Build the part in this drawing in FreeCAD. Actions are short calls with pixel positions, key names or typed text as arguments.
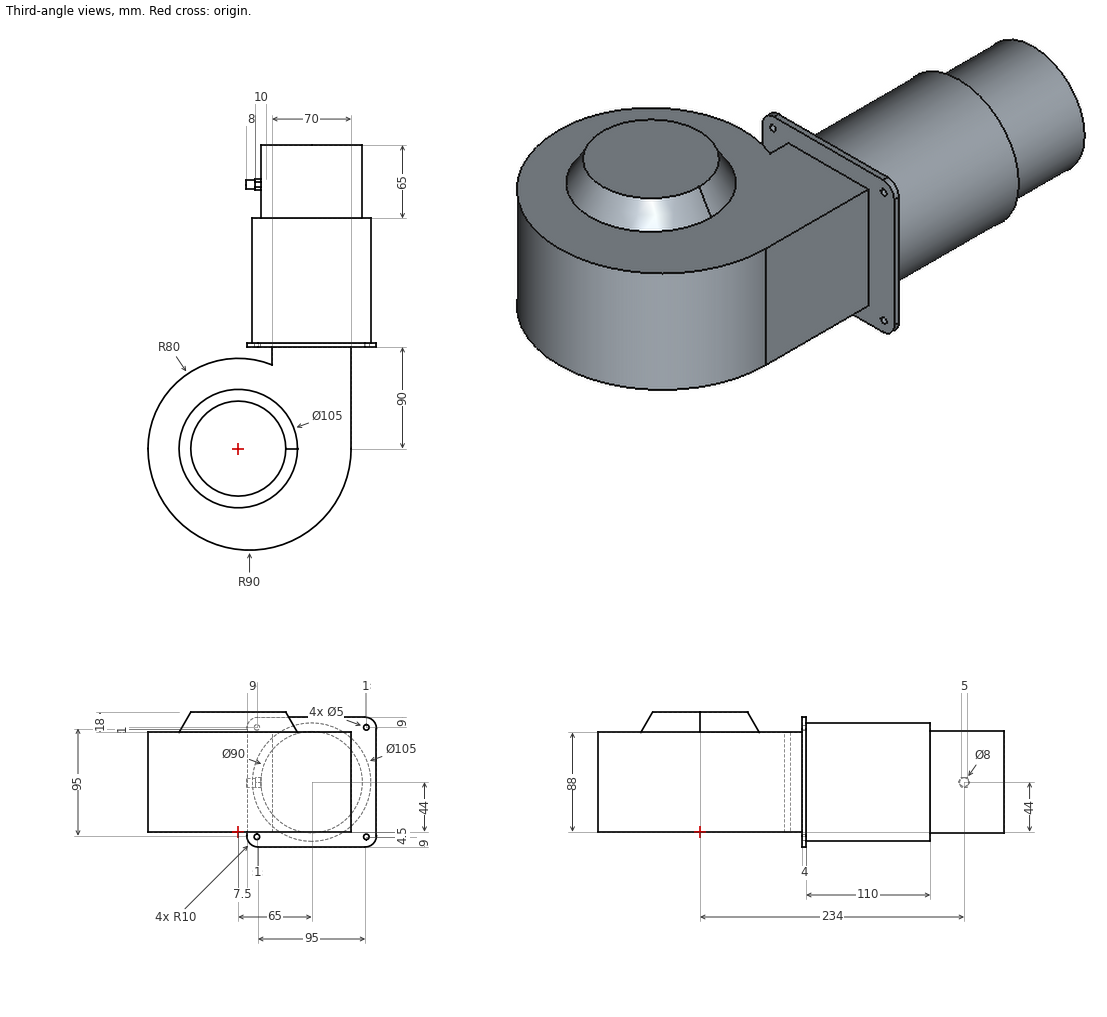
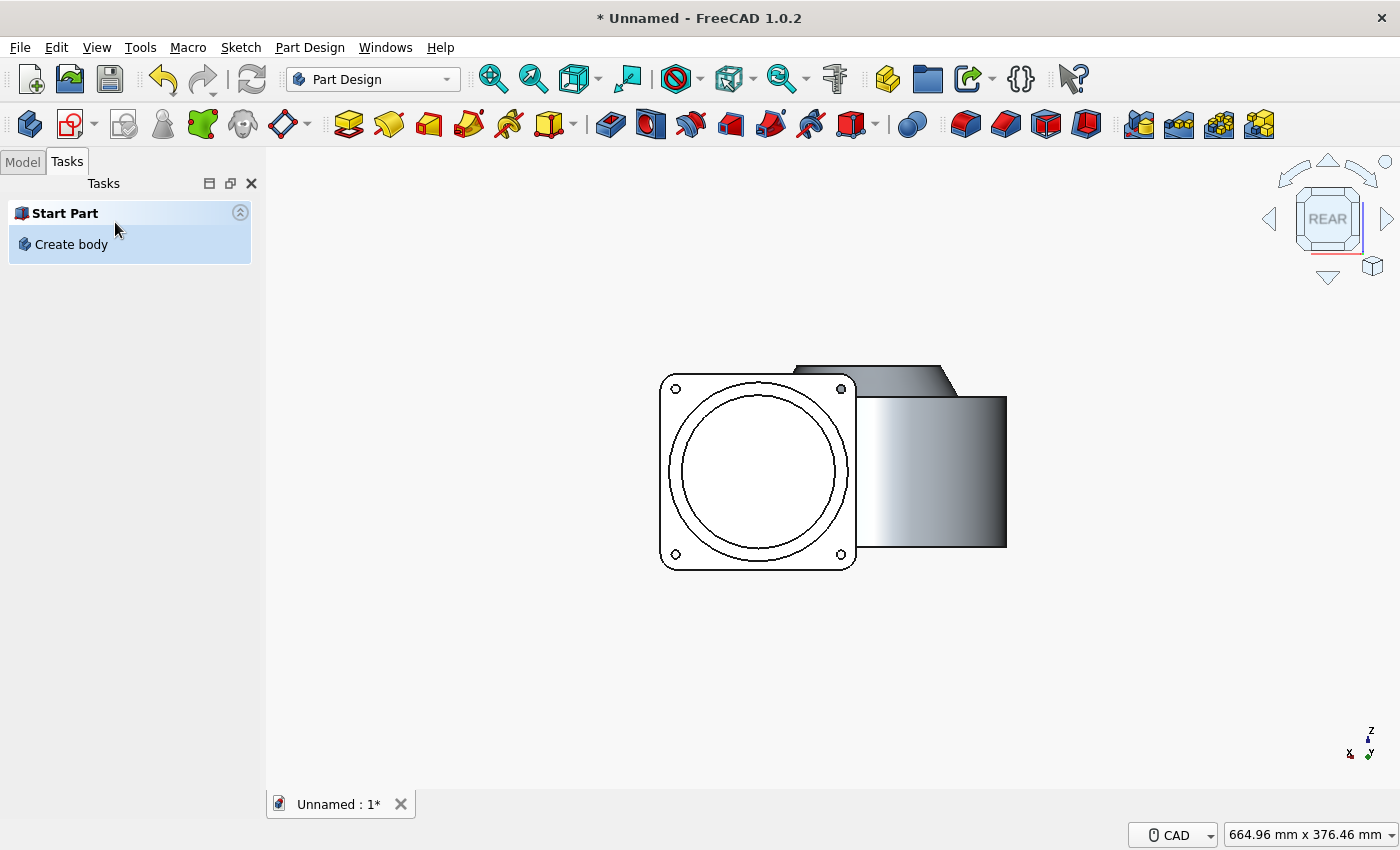
key(v)
key(f)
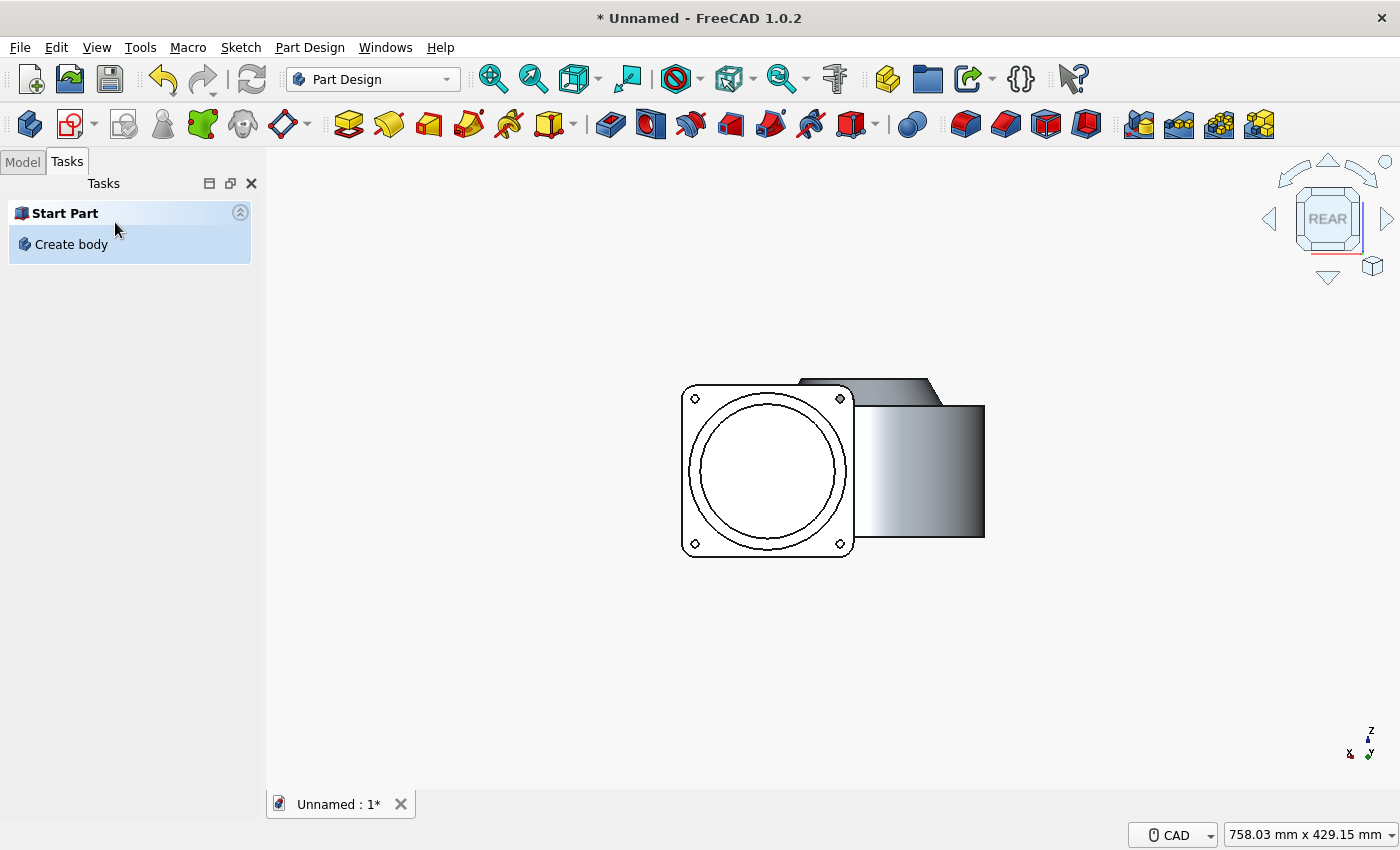
click(30, 124)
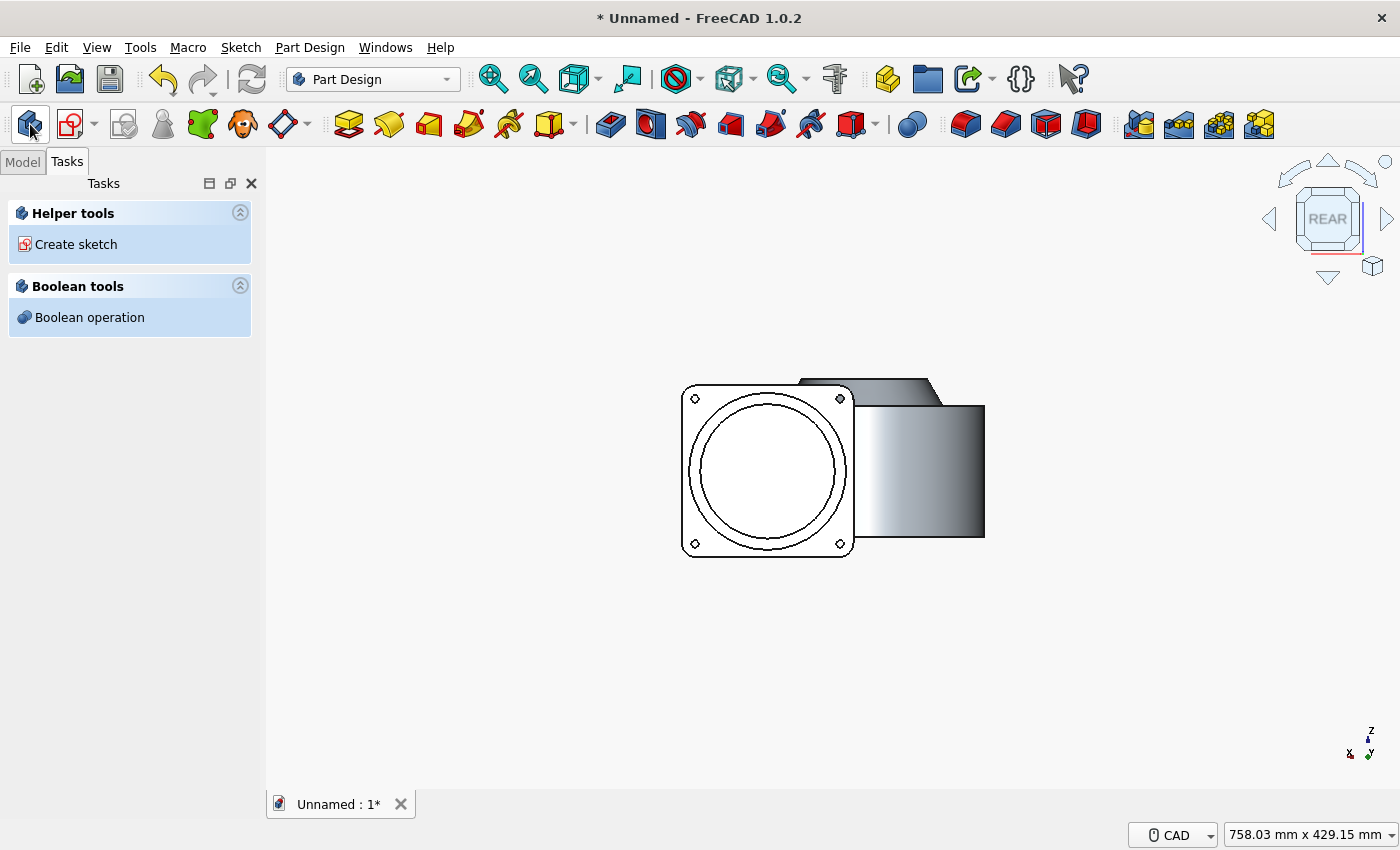
click(23, 161)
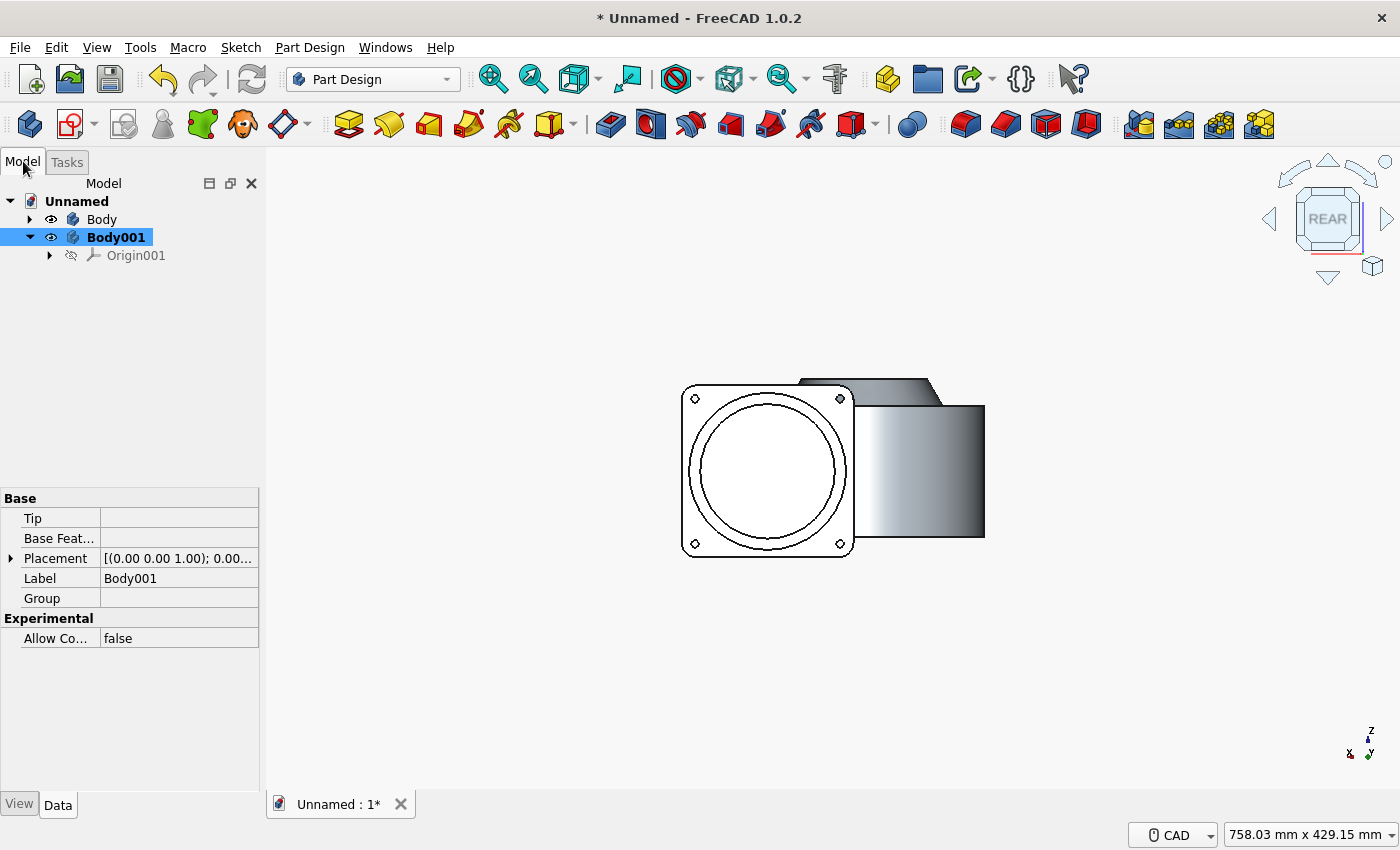
click(50, 255)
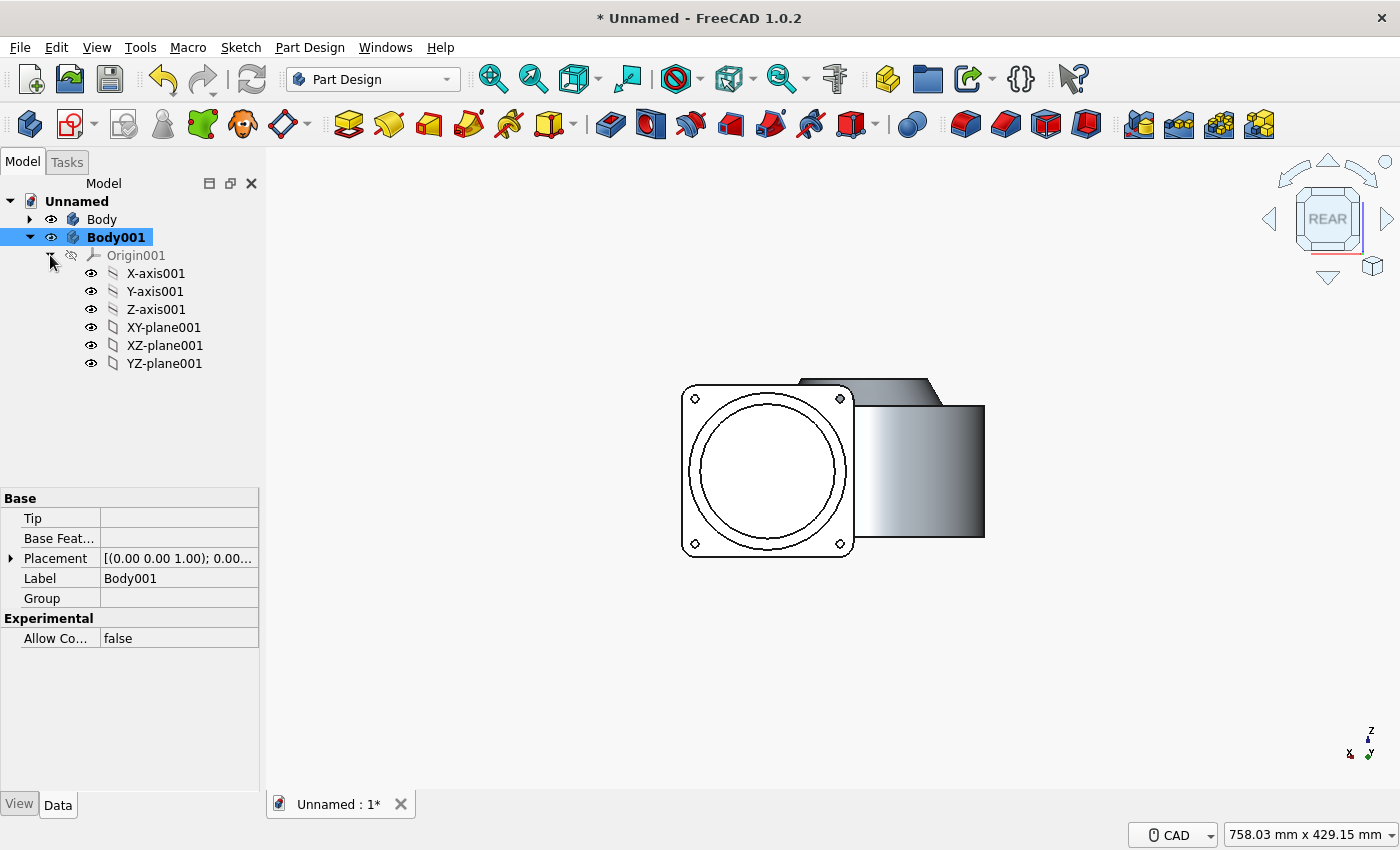
click(136, 363)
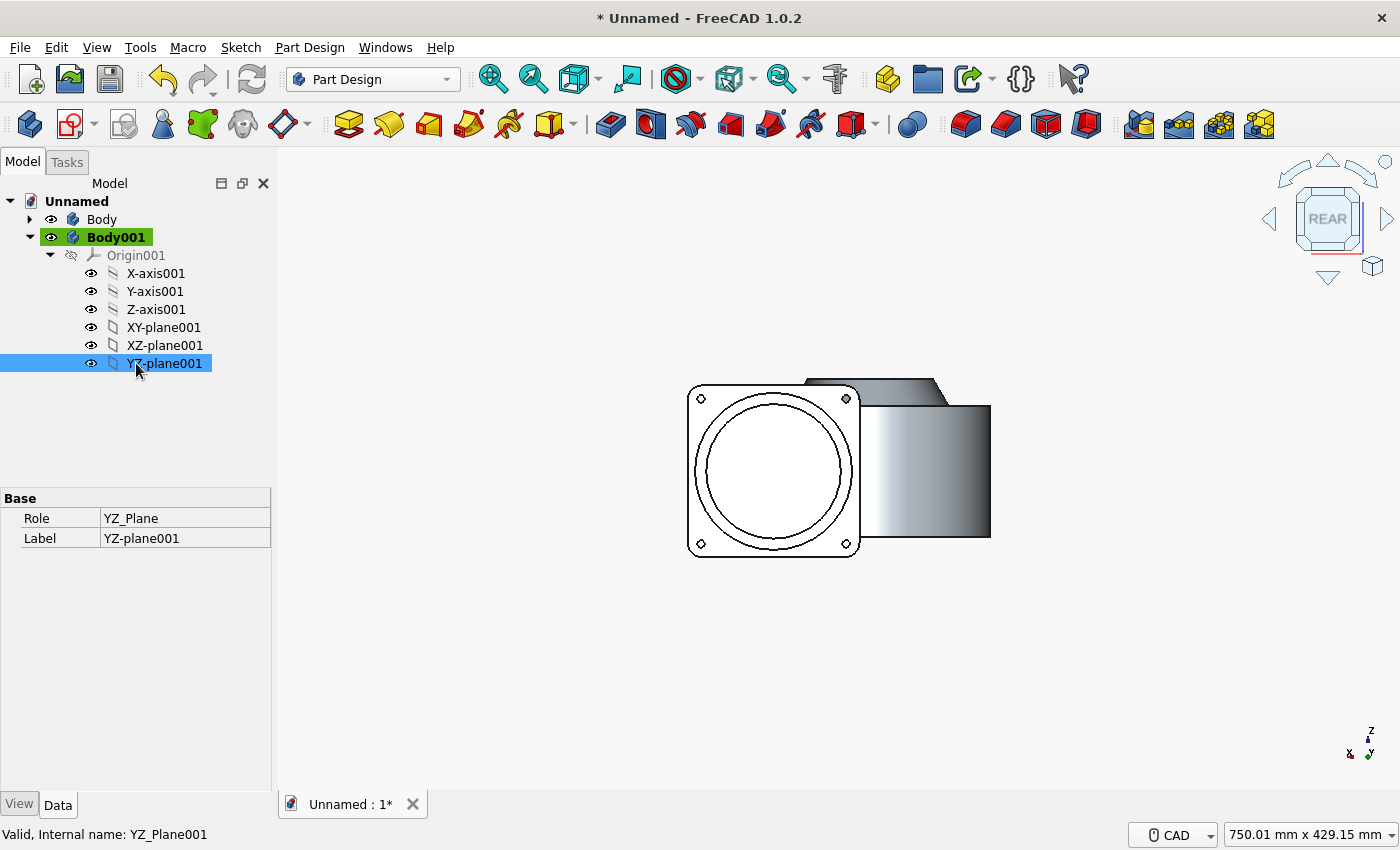
click(284, 124)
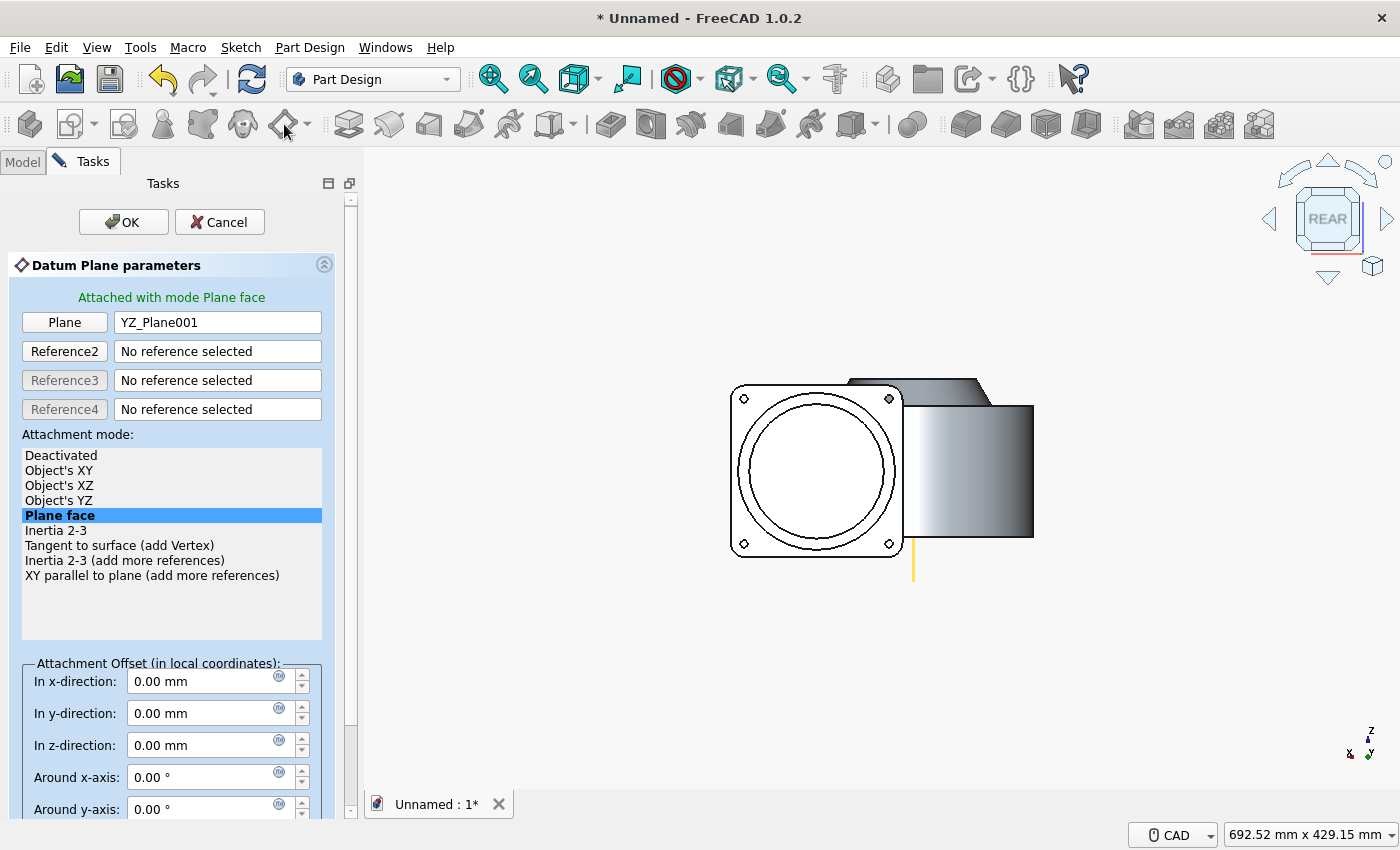
triple_click(210, 745)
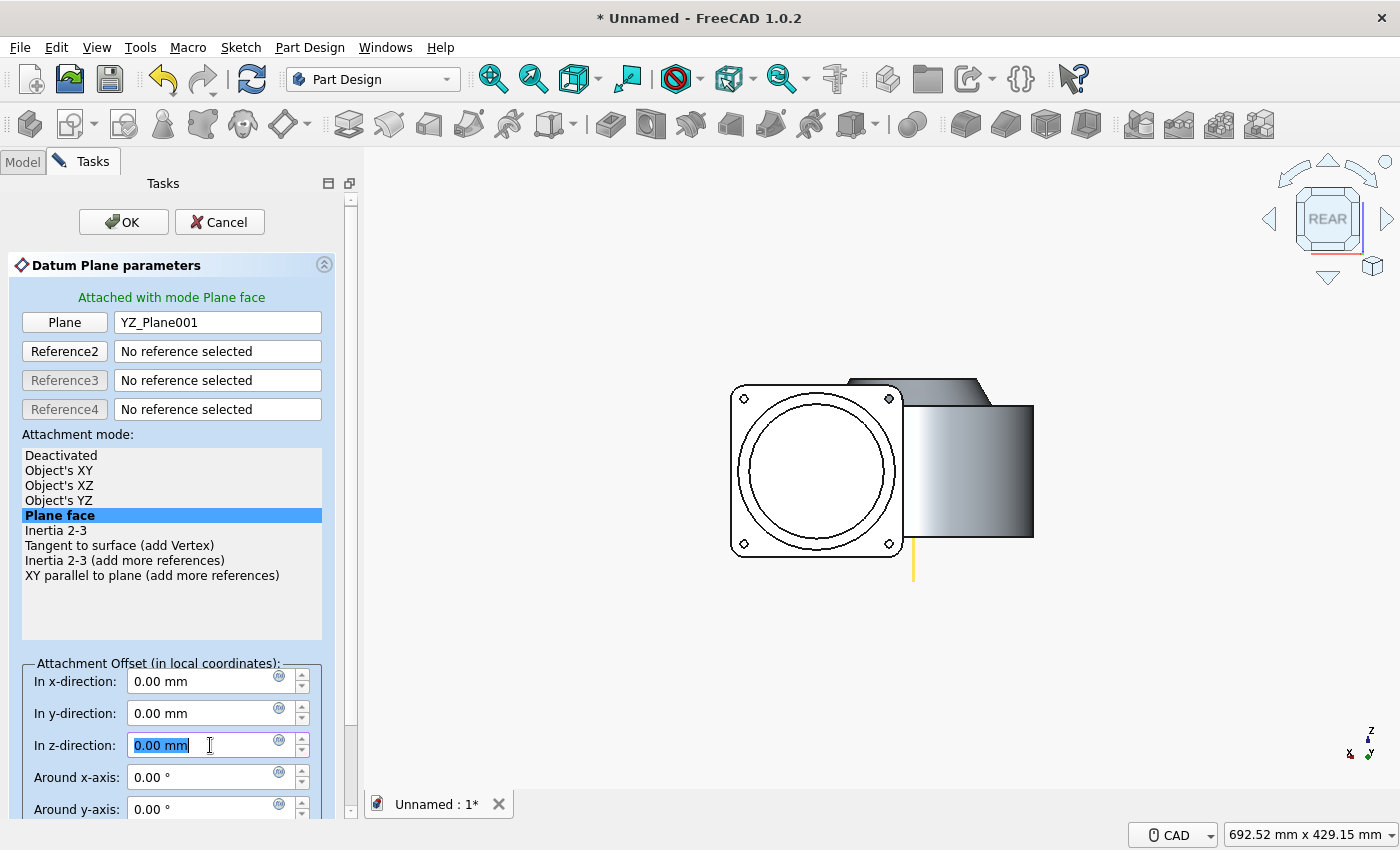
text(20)
key(Tab)